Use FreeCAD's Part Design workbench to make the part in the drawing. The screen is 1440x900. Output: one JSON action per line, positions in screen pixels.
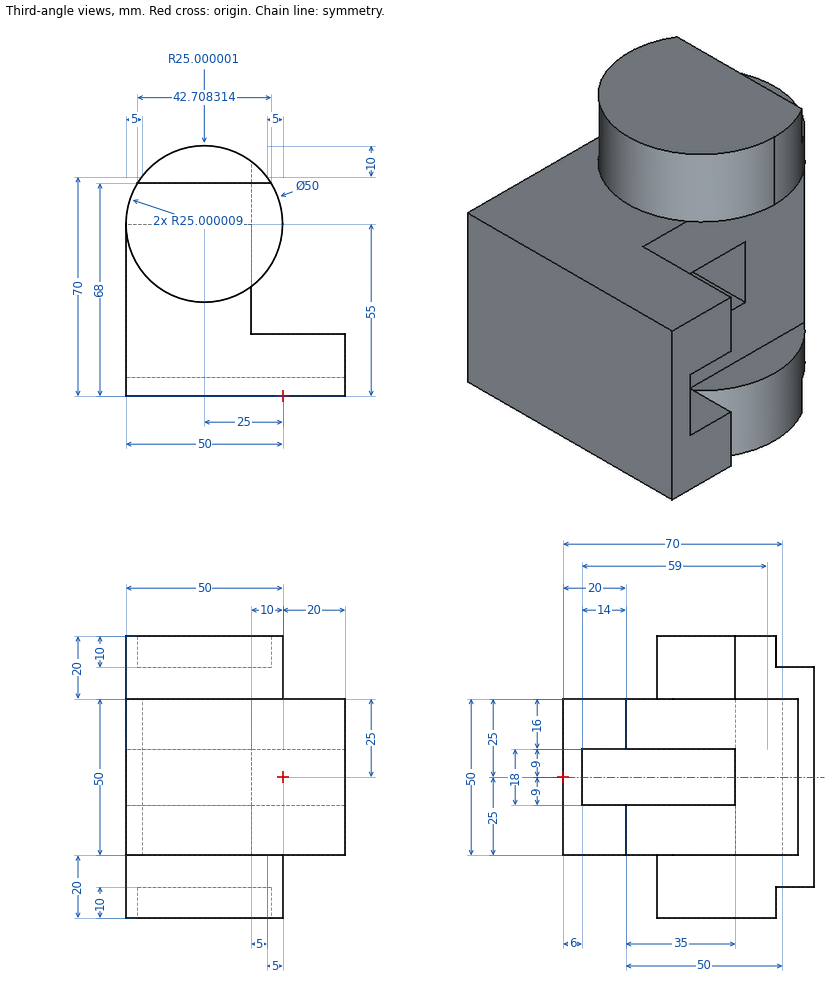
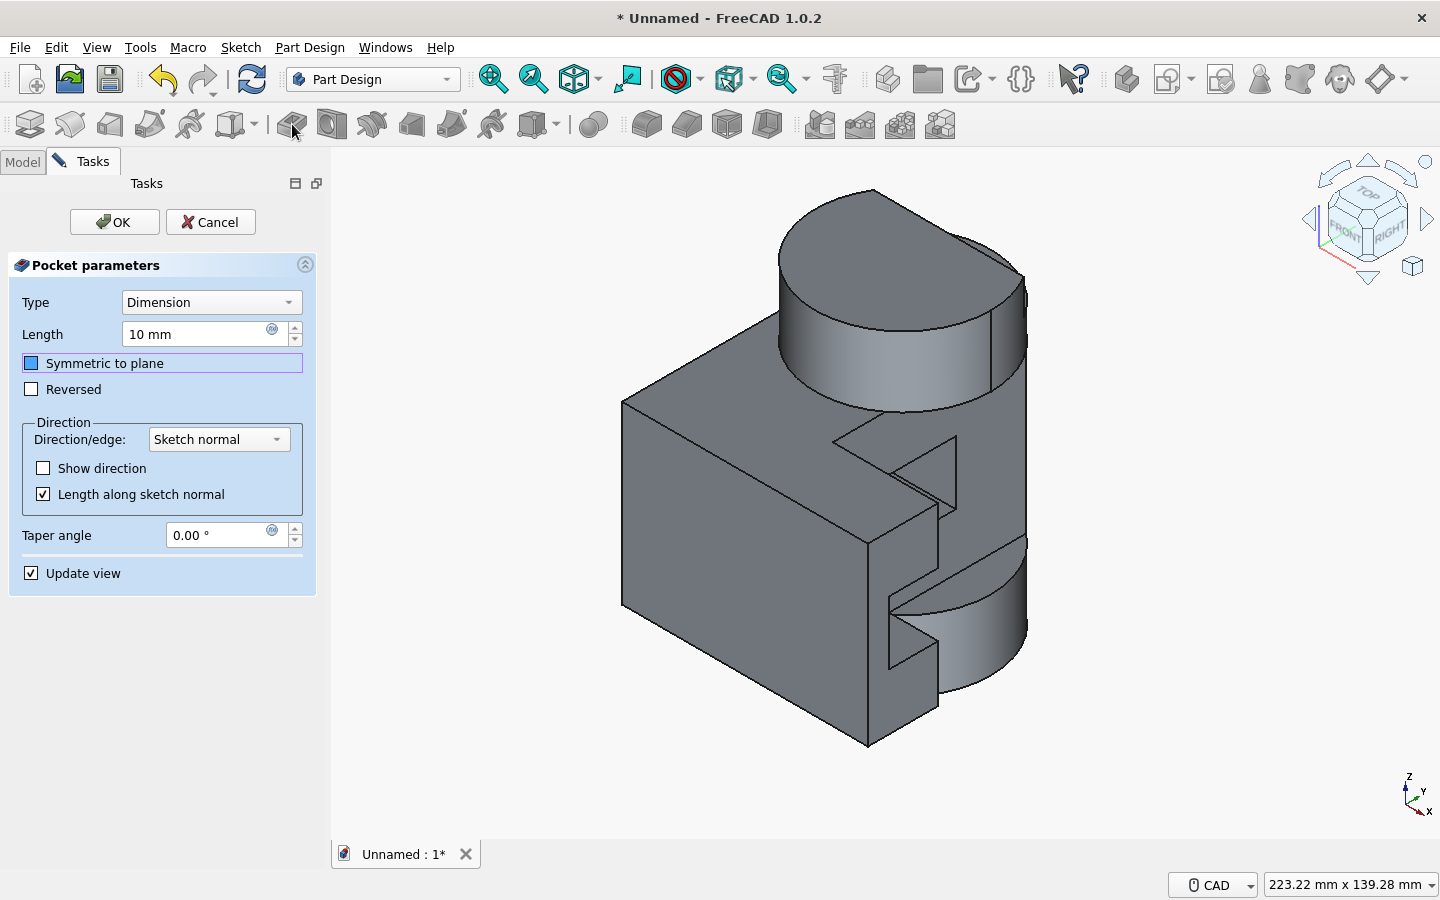
{"action": "left_click", "coordinate": [115, 222]}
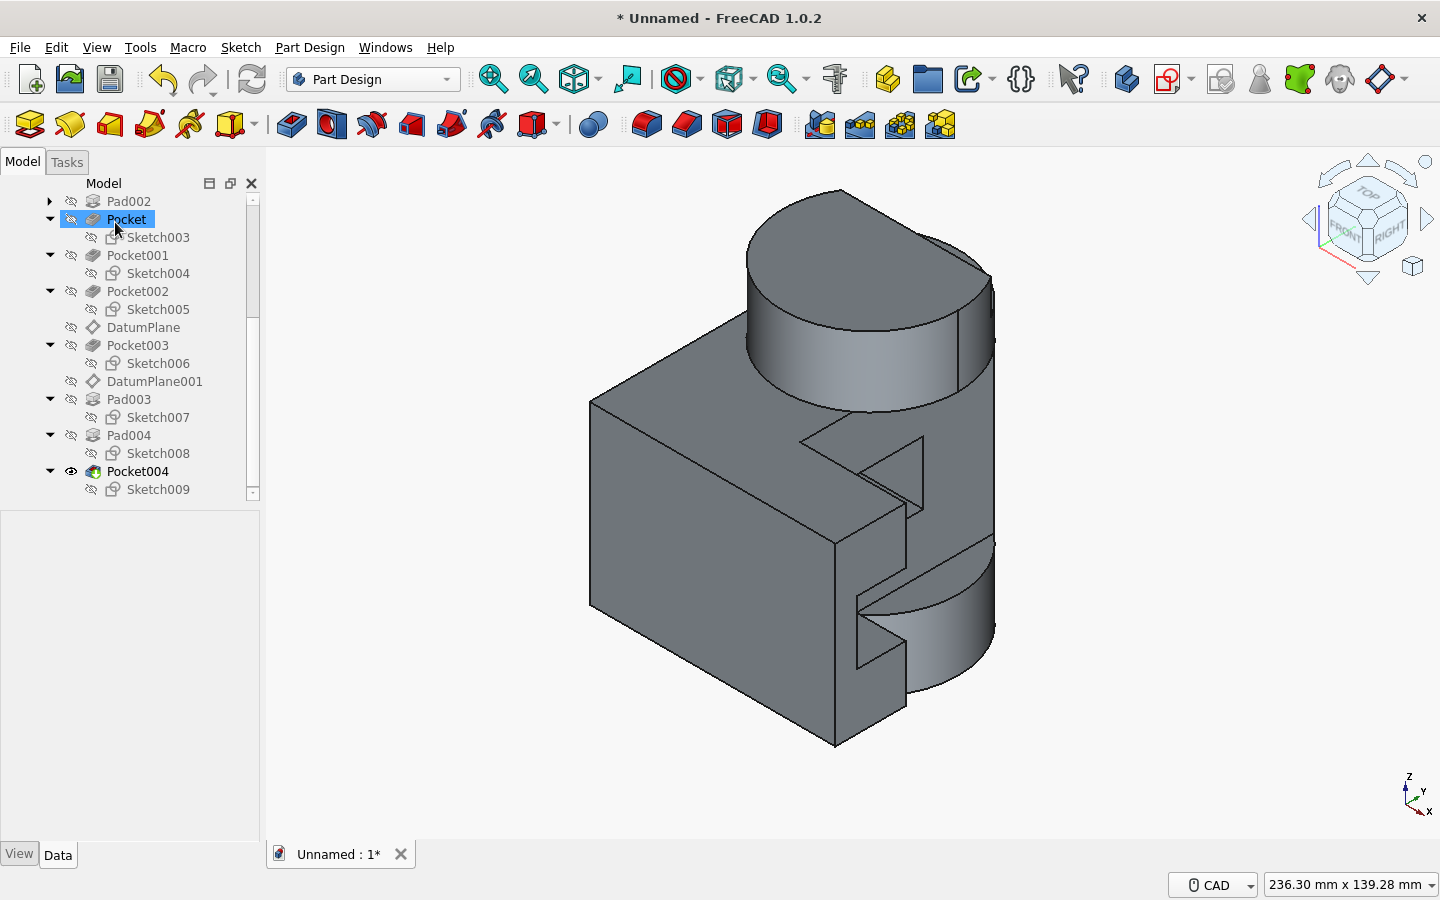
{"action": "scroll", "coordinate": [140, 341], "scroll_direction": "down", "scroll_amount": 3}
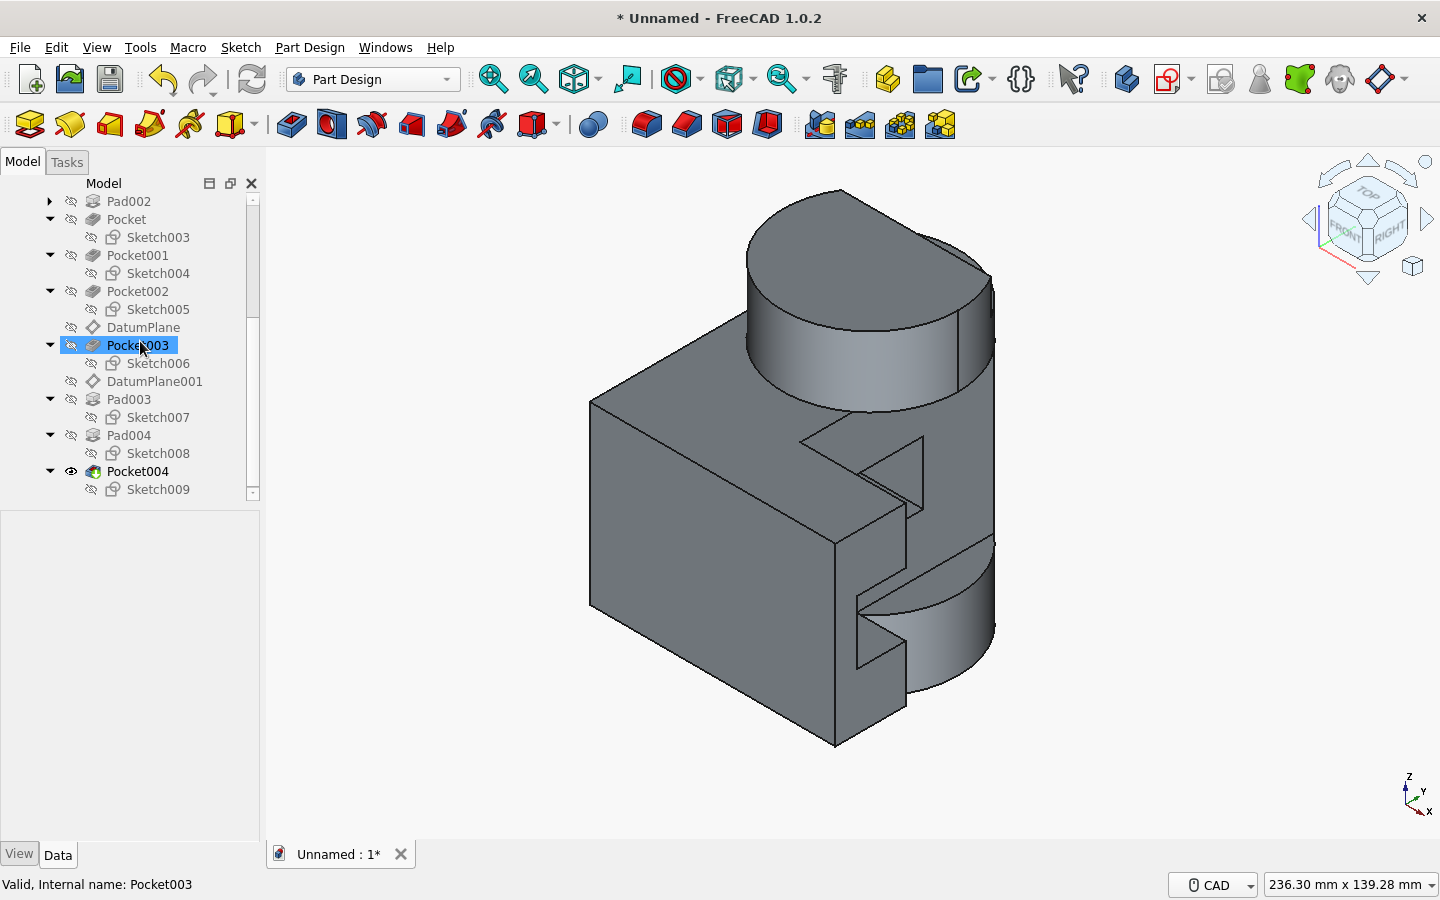
{"action": "scroll", "coordinate": [140, 341], "scroll_direction": "up", "scroll_amount": 15}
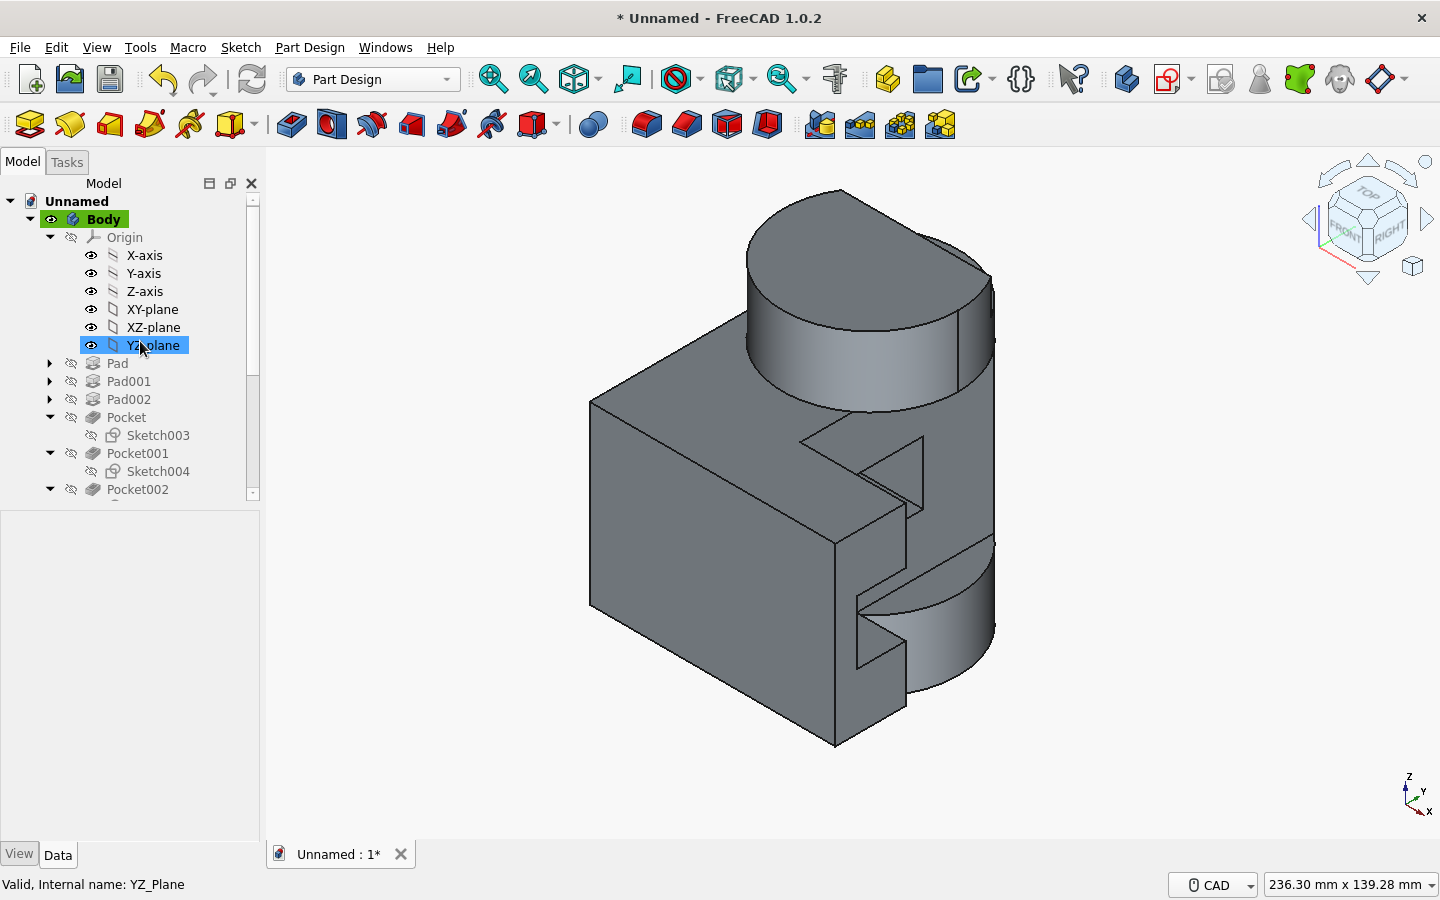
{"action": "left_click", "coordinate": [136, 309]}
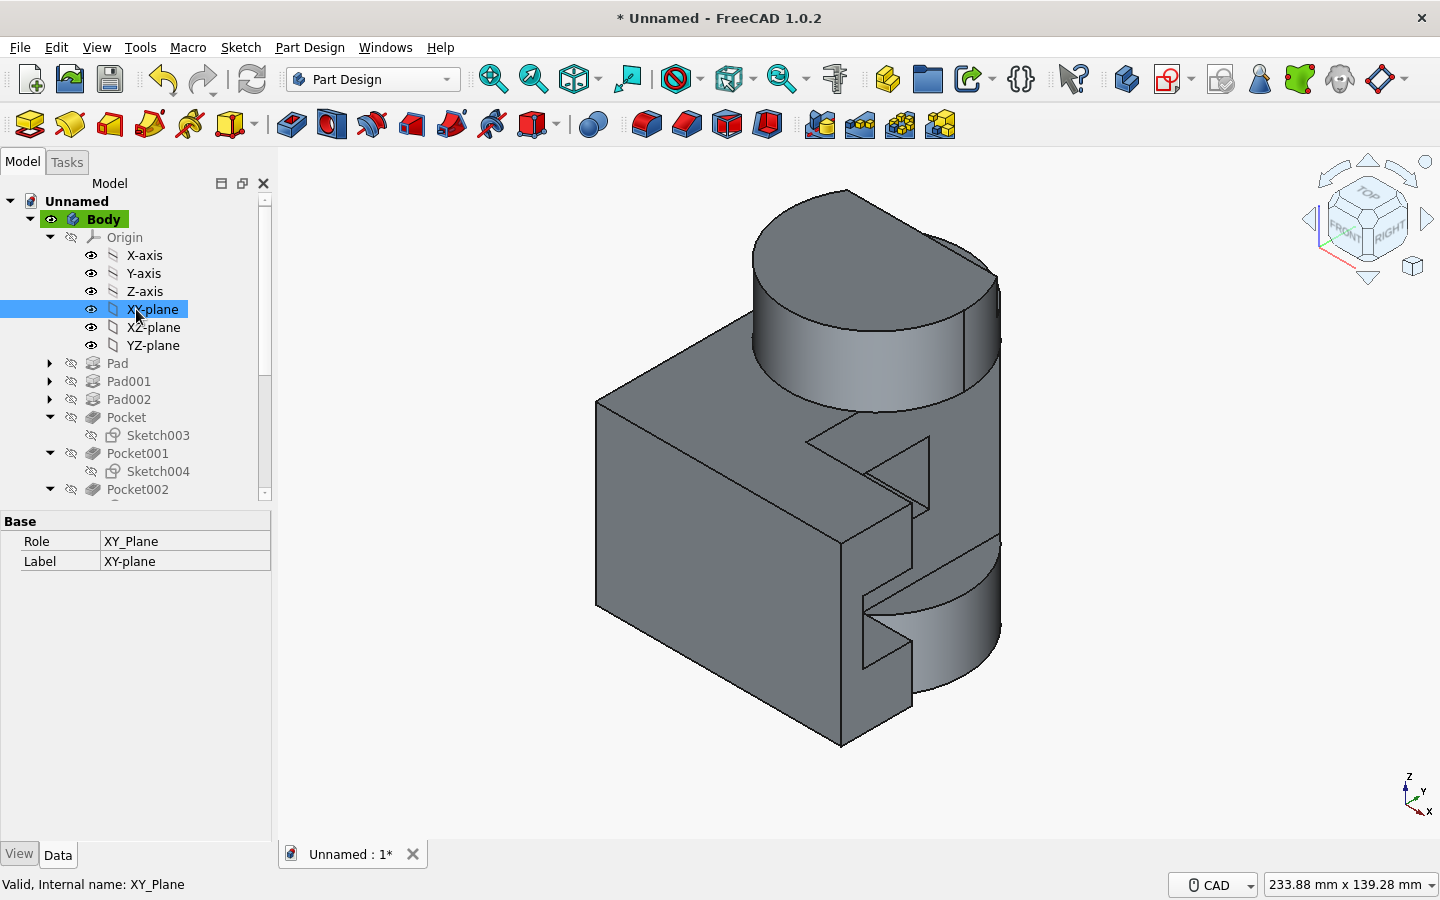
{"action": "left_click", "coordinate": [1380, 80]}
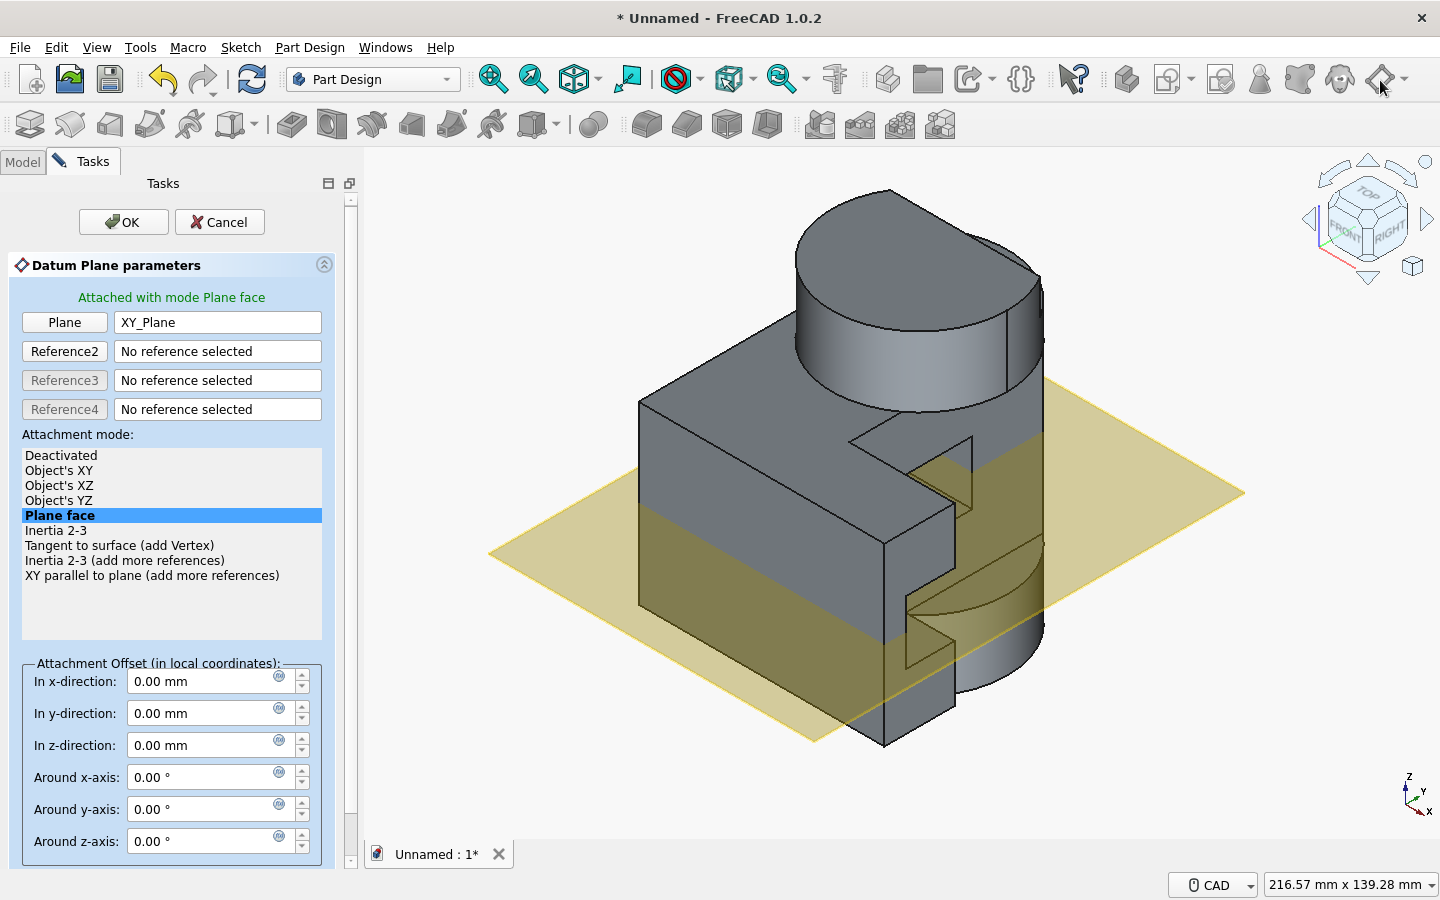
{"action": "triple_click", "coordinate": [210, 745]}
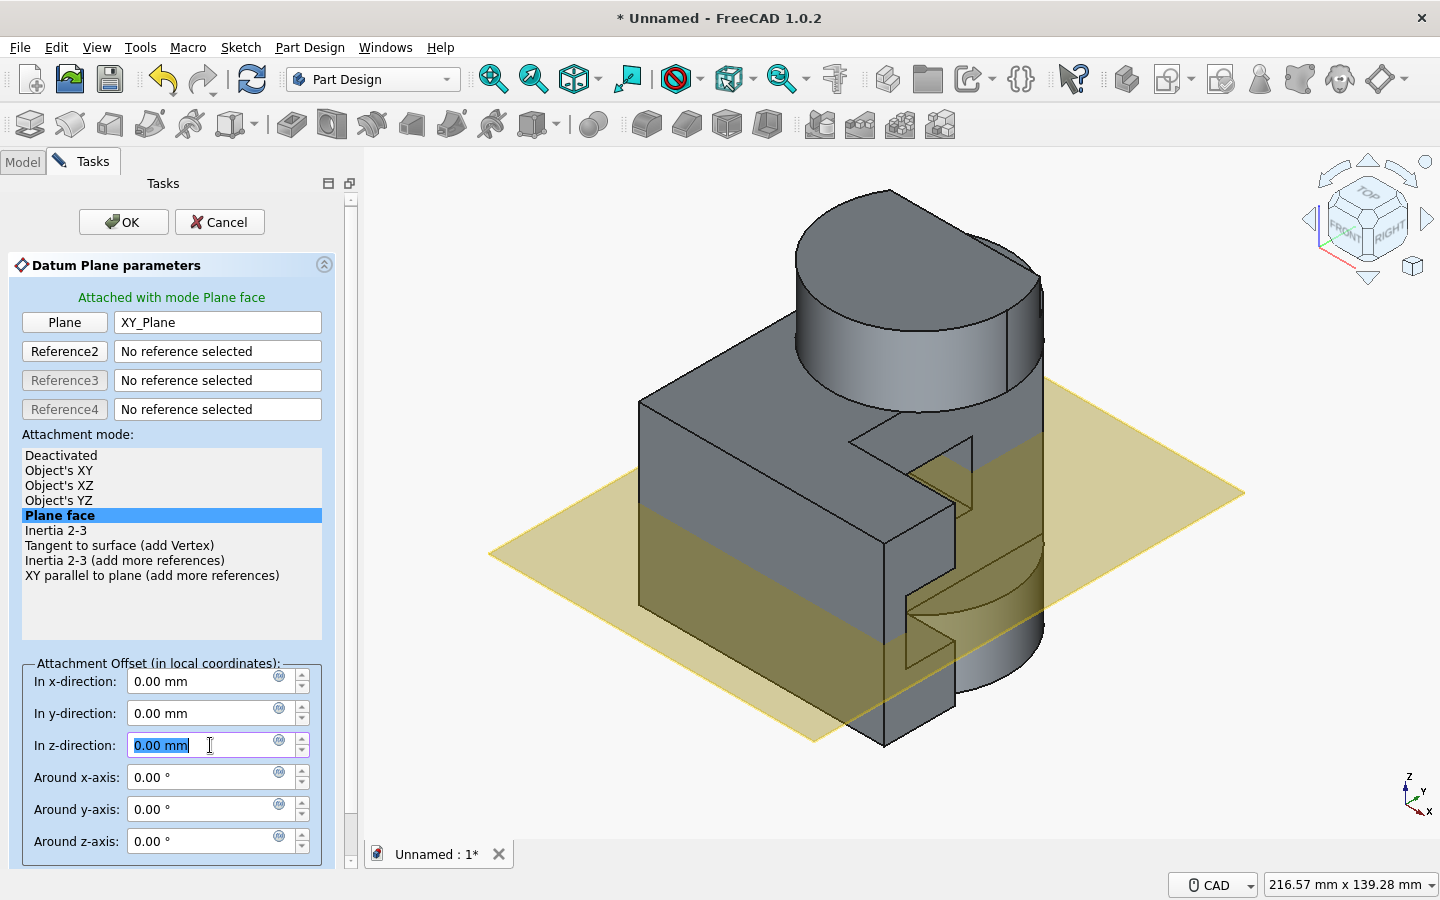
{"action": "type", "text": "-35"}
{"action": "key", "text": "Tab"}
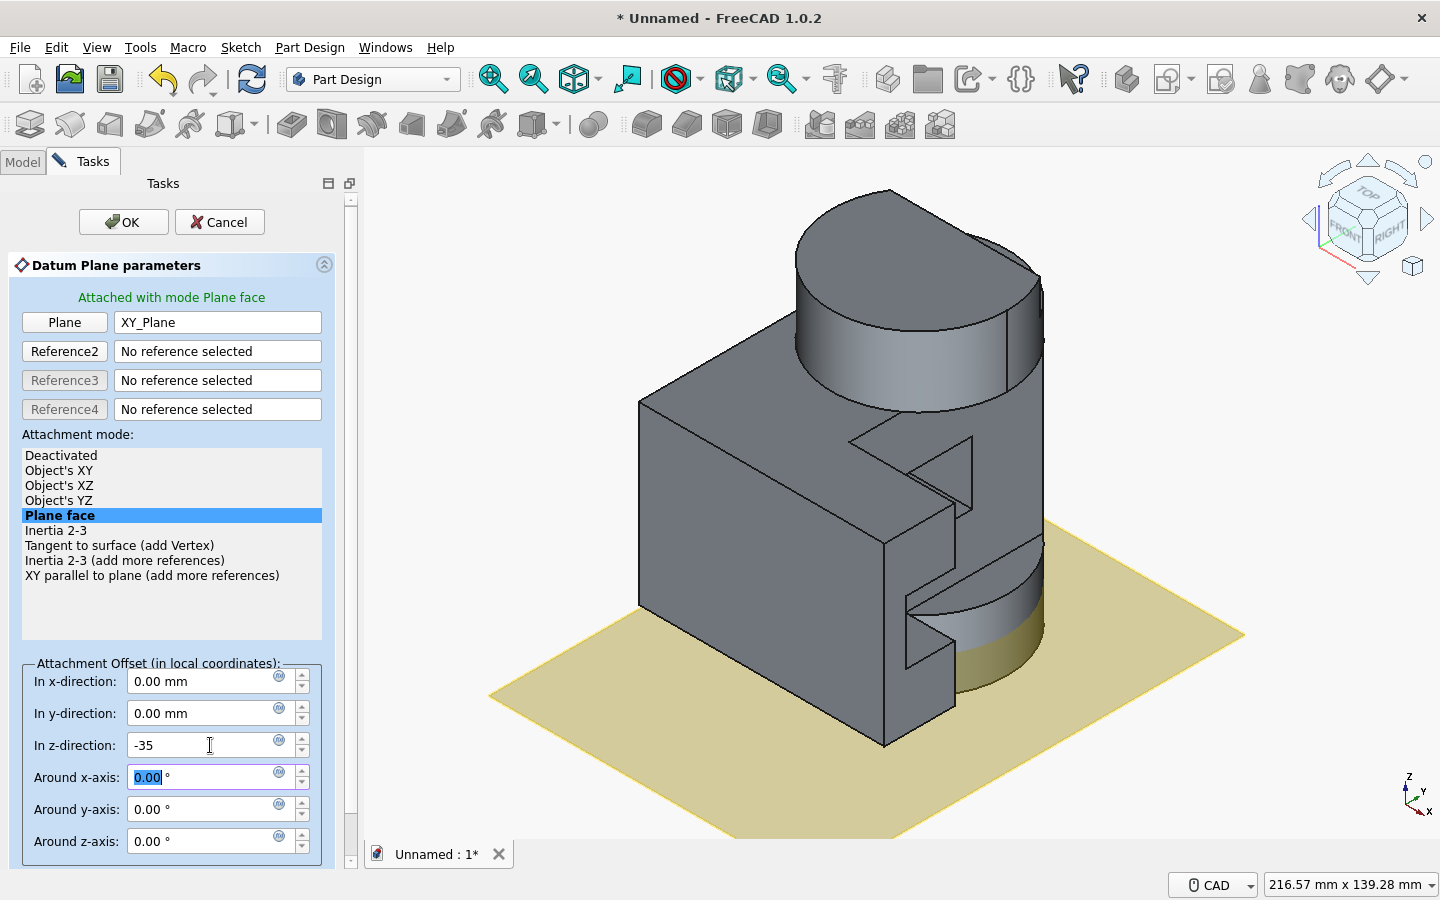
{"action": "left_click", "coordinate": [124, 222]}